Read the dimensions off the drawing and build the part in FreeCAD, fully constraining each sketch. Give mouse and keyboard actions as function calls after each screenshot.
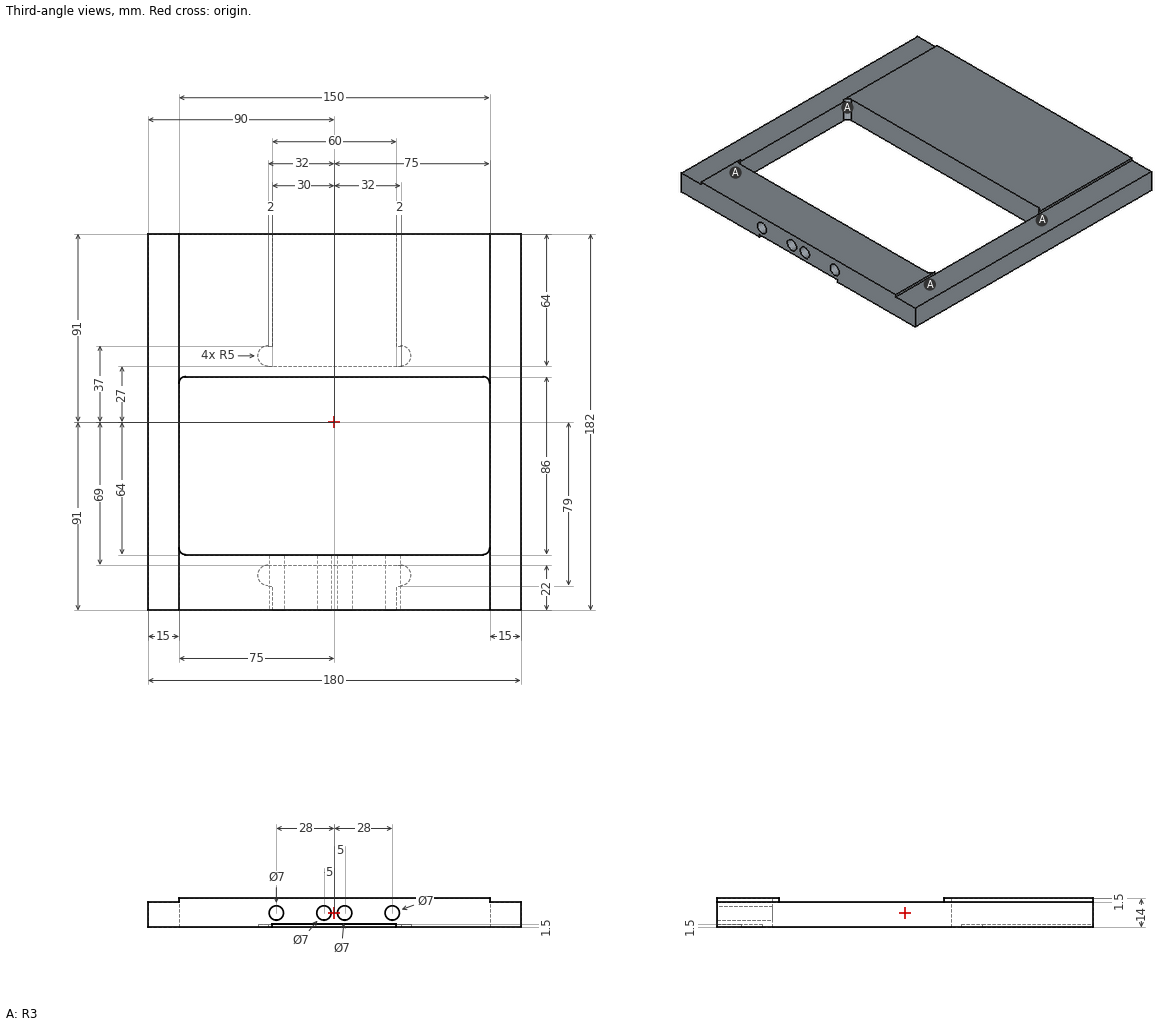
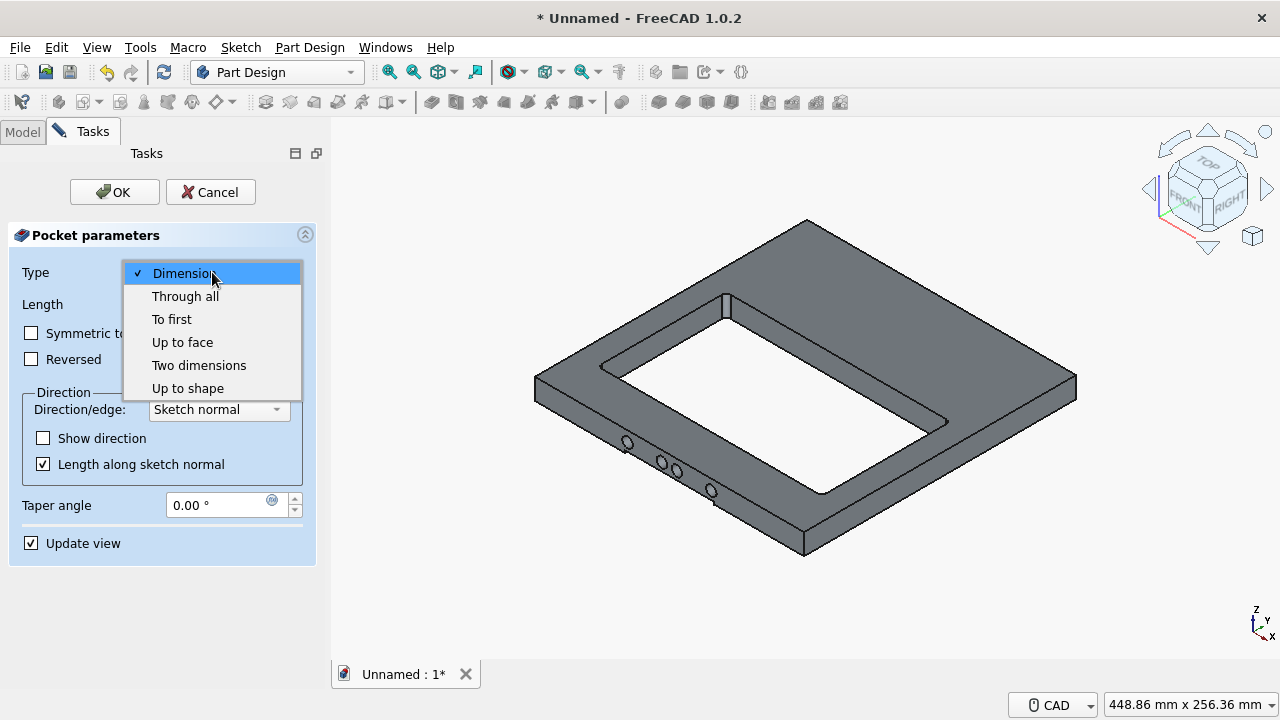
click(212, 320)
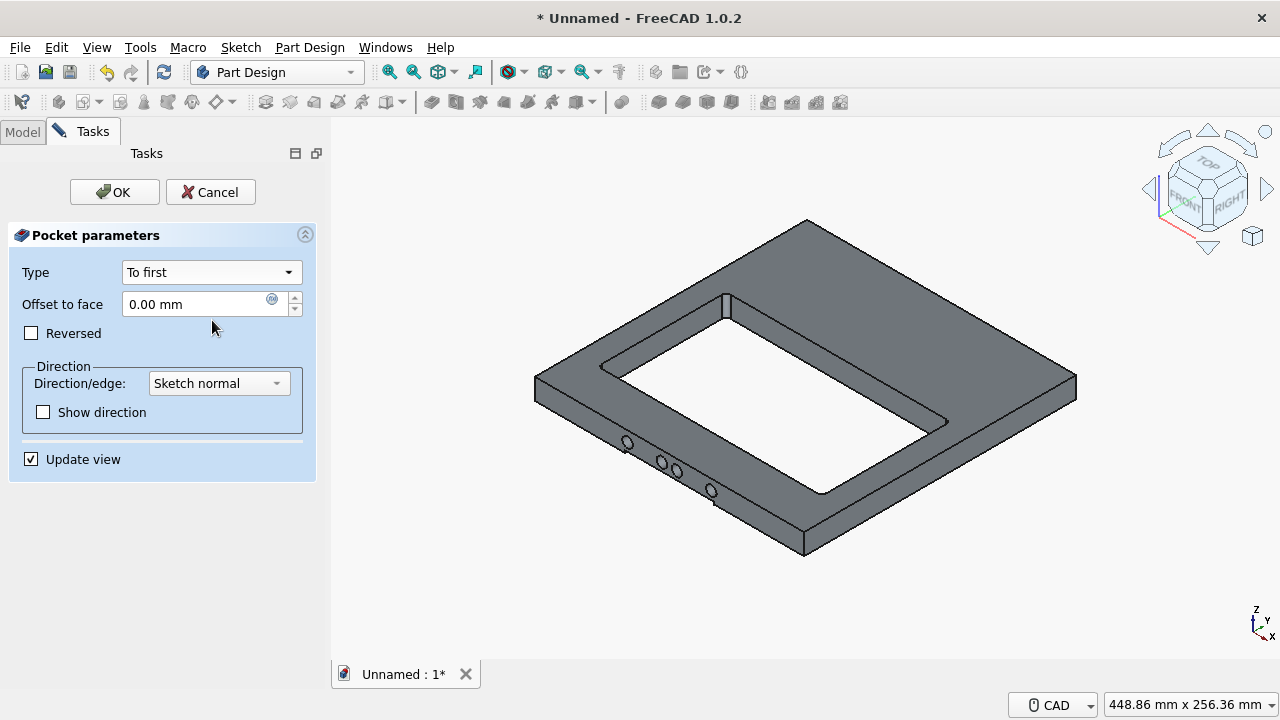
click(115, 192)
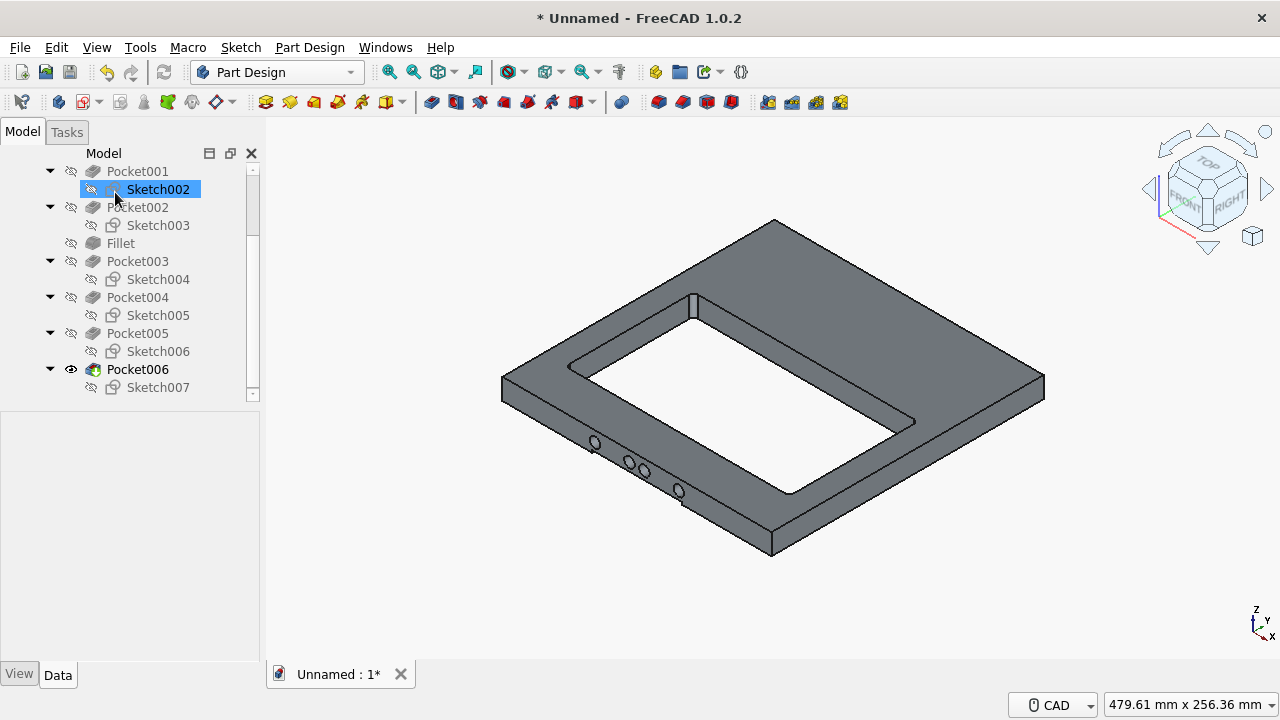
click(928, 374)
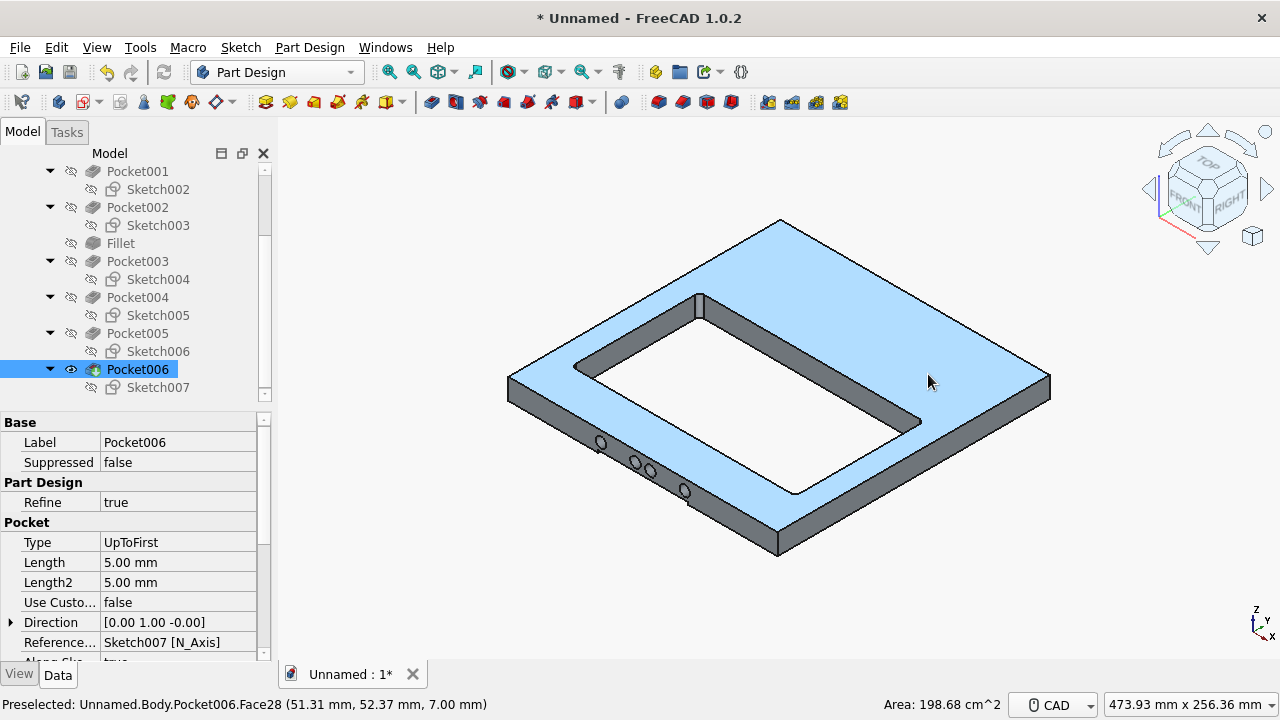
click(84, 102)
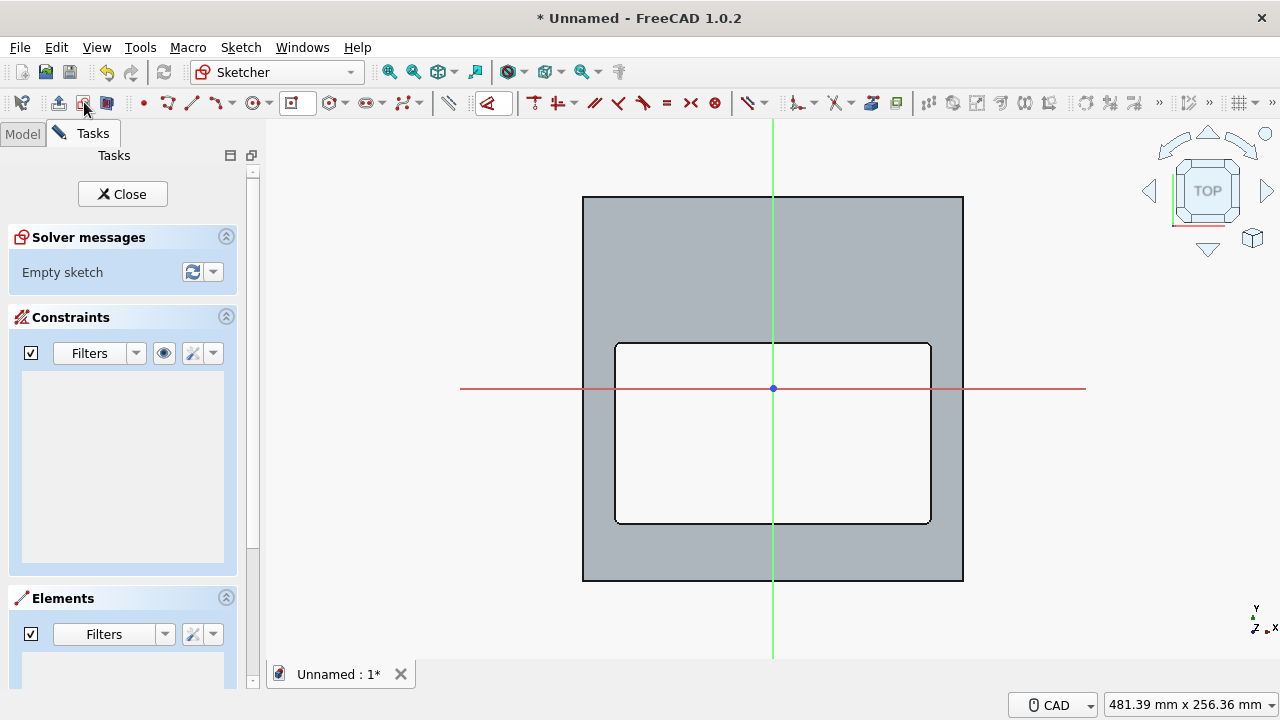
key(g)
key(r)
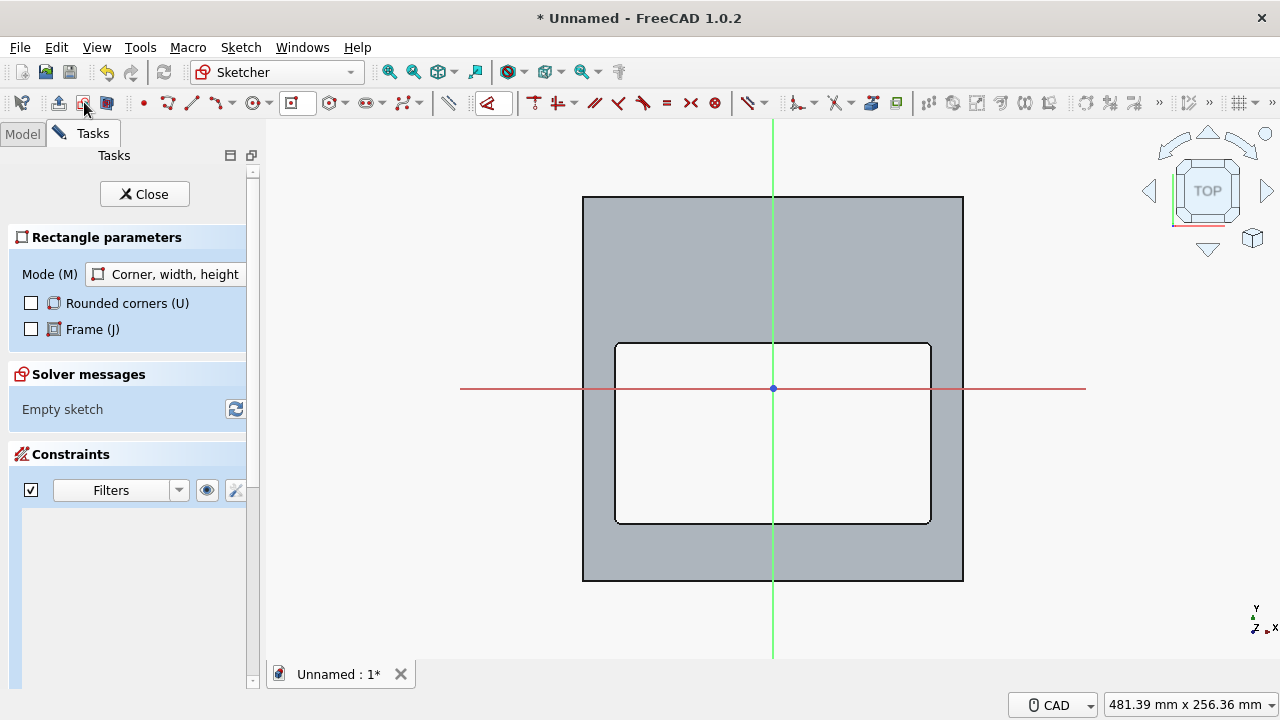
click(583, 197)
move(615, 581)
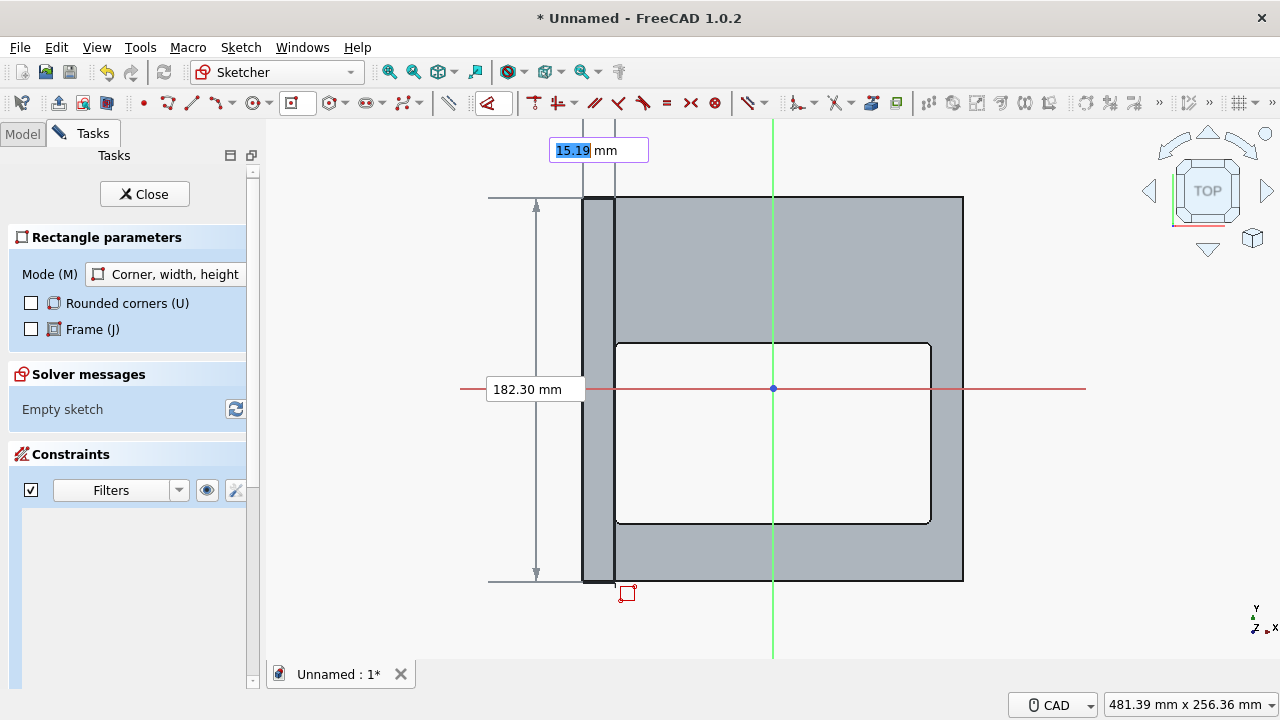
text(15)
key(Tab)
text(182)
key(Return)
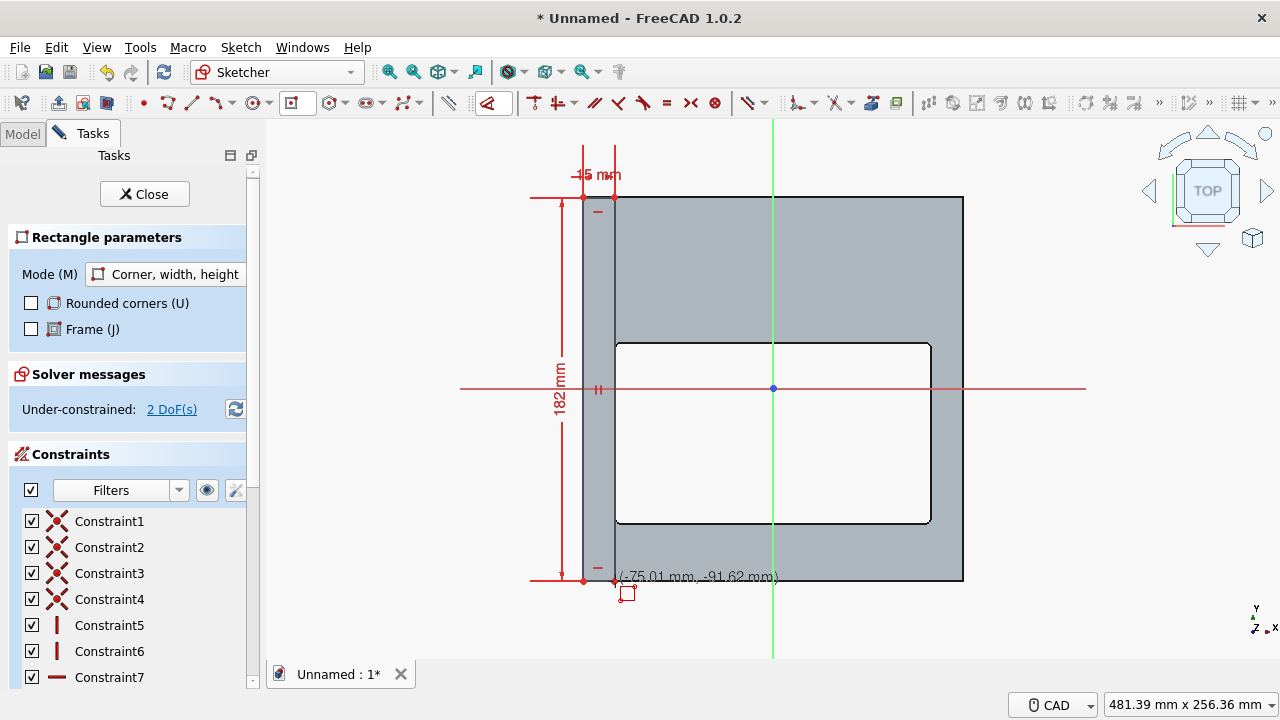
click(931, 197)
move(963, 581)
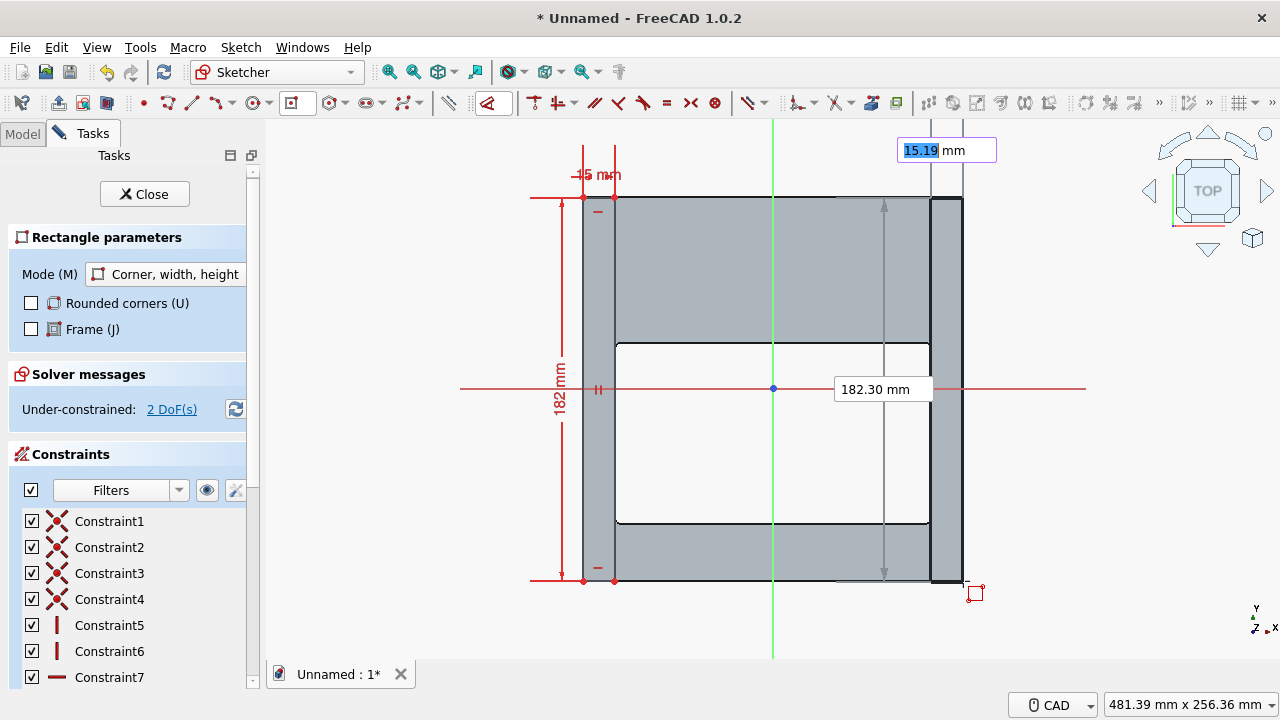
text(15)
key(Tab)
text(182)
key(Return)
key(Escape)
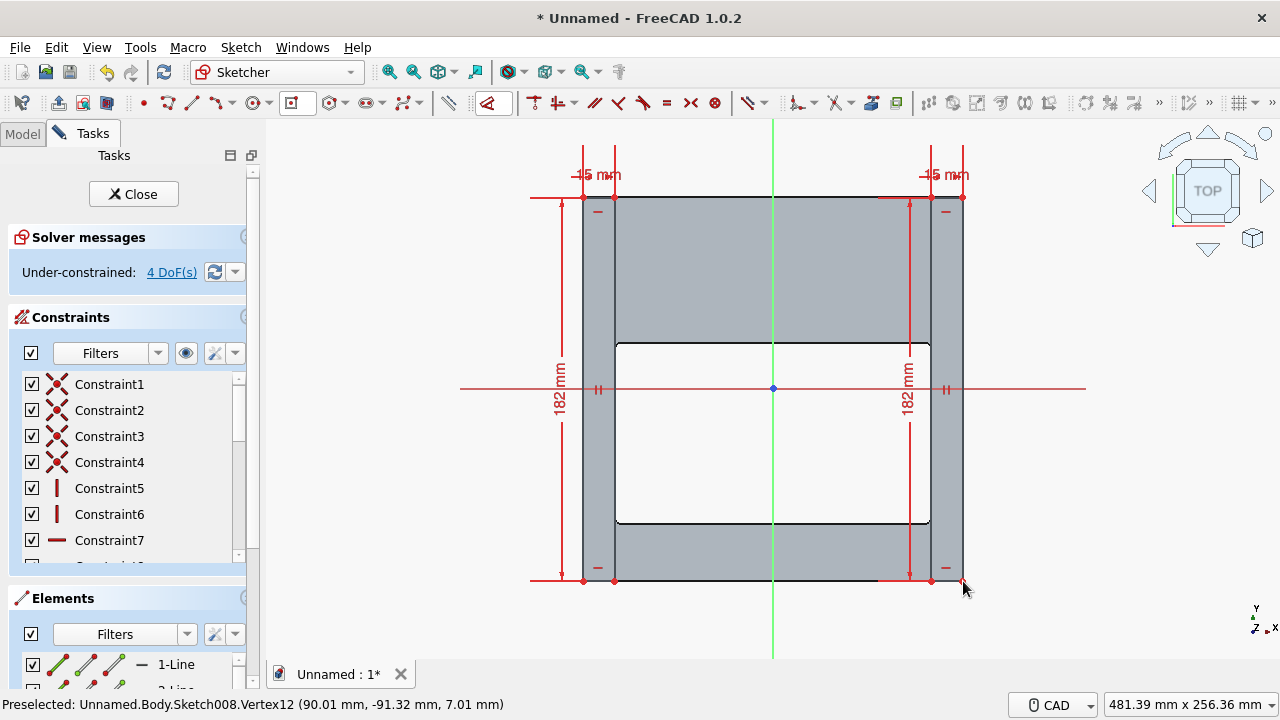
click(583, 198)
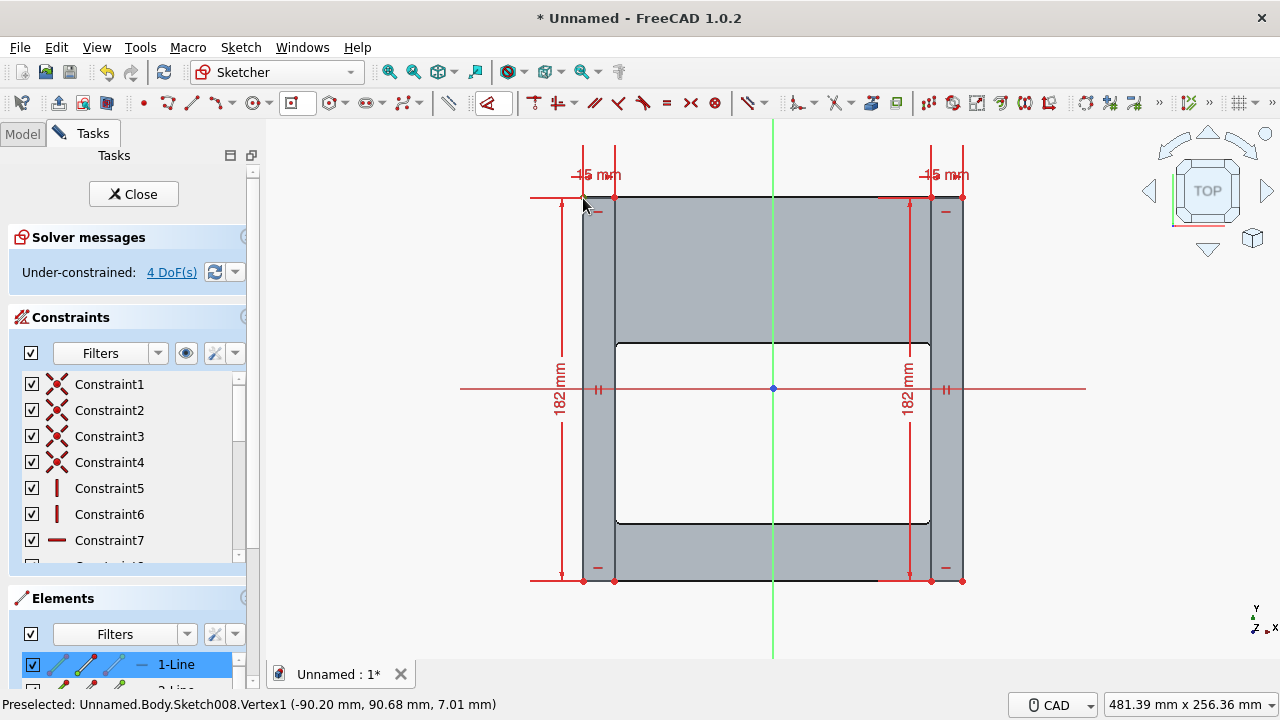
key(l)